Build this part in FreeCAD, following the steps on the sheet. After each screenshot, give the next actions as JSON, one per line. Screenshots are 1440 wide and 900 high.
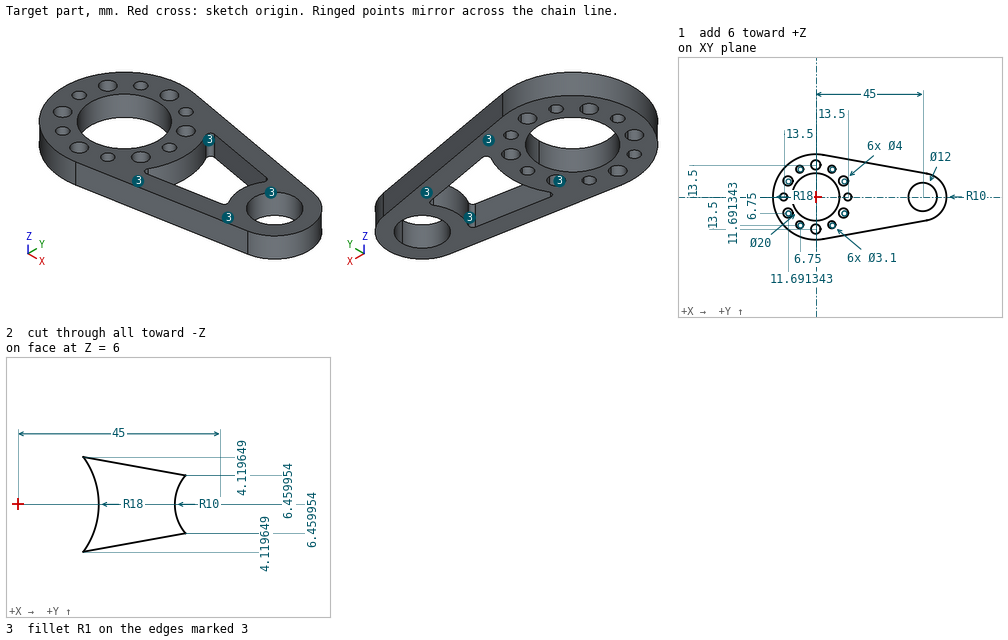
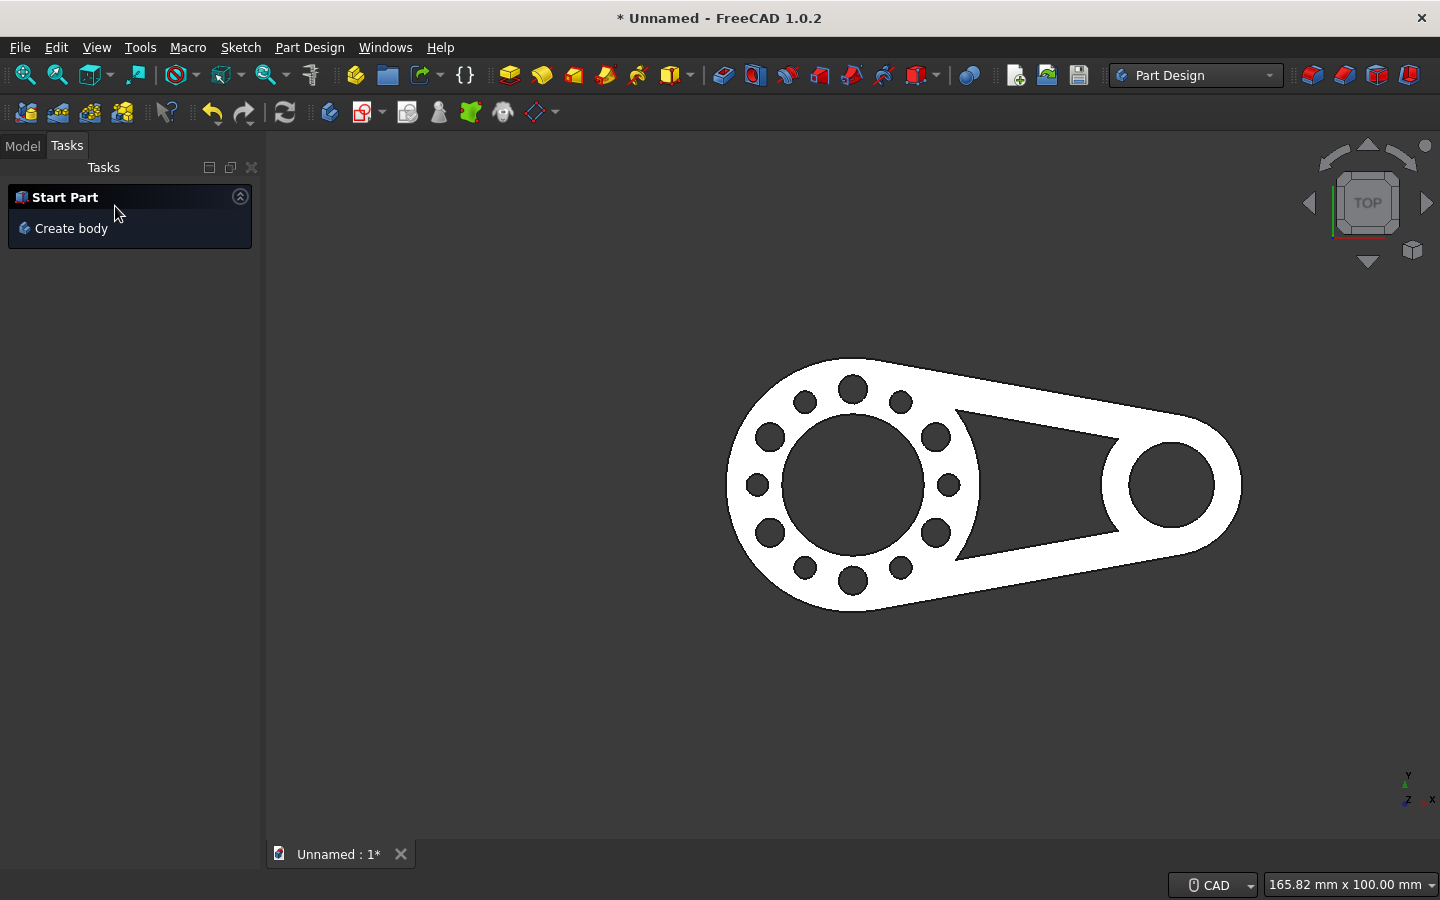
{"action": "left_click", "coordinate": [26, 76]}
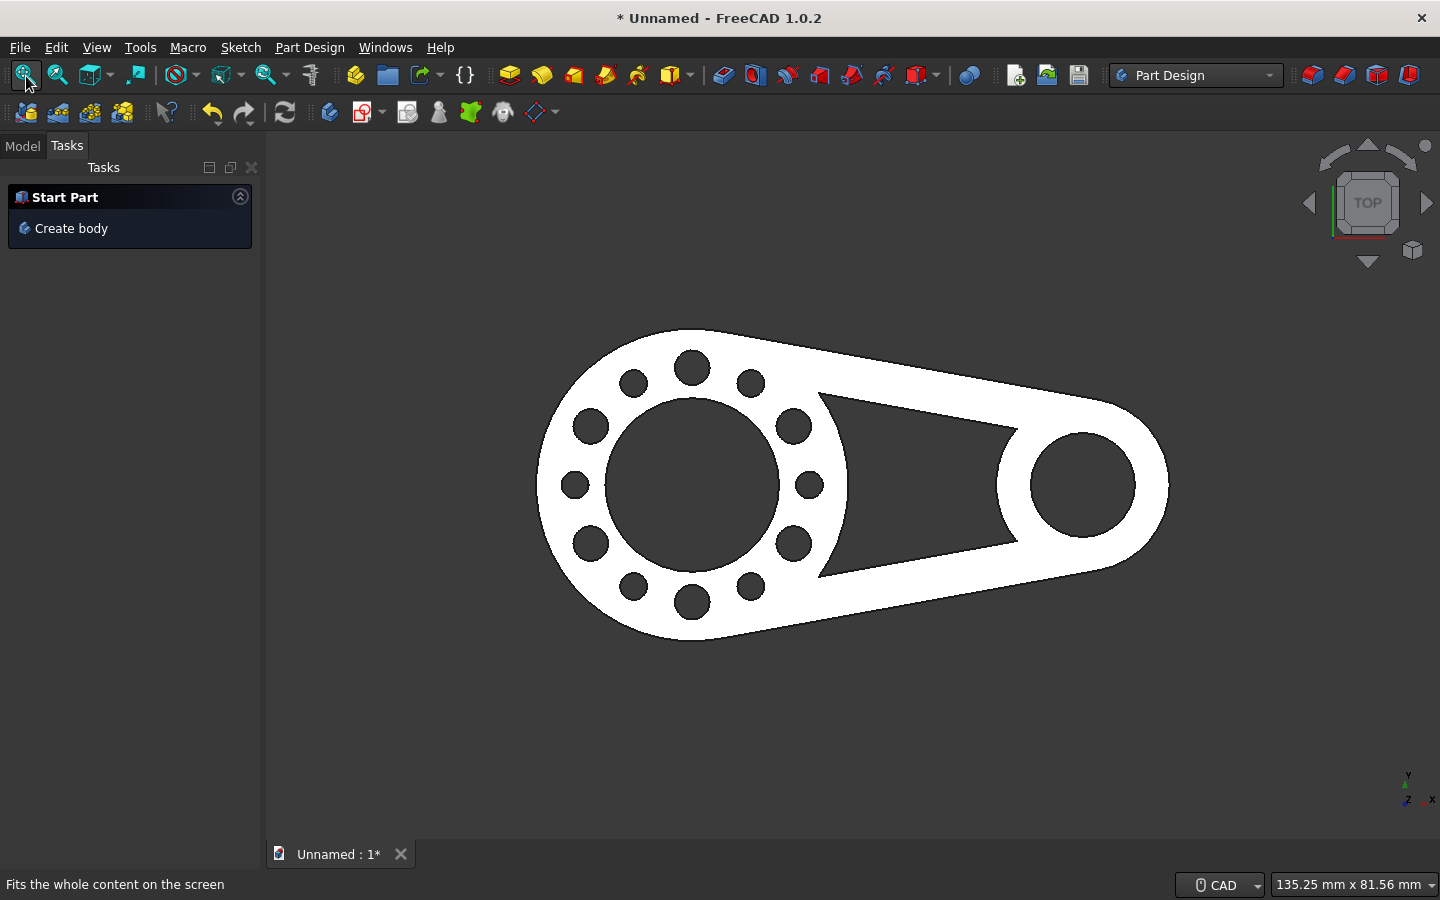
{"action": "key", "text": "1"}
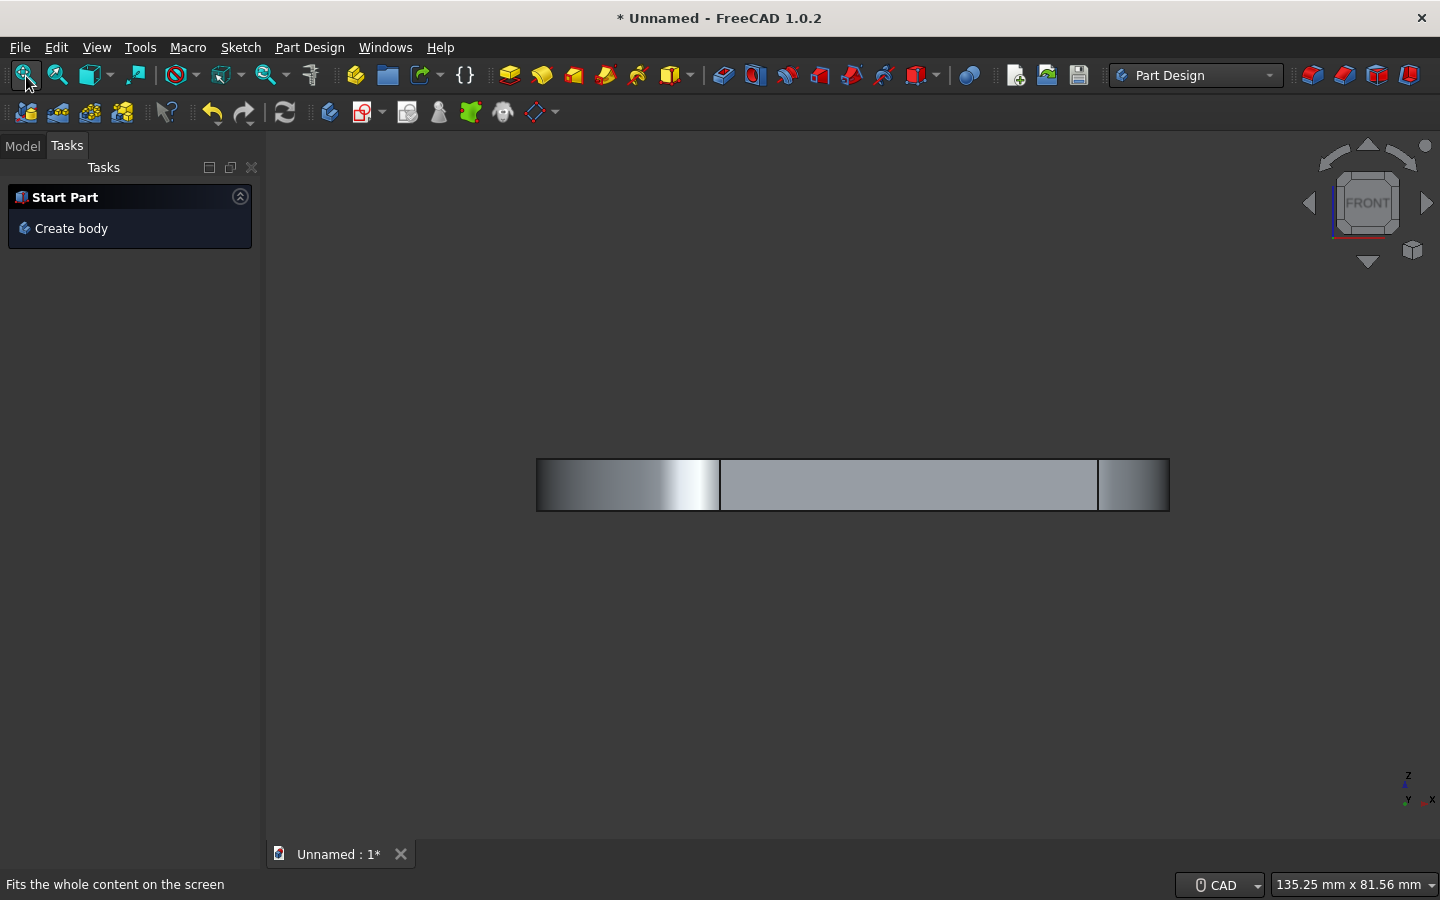
{"action": "key", "text": "3"}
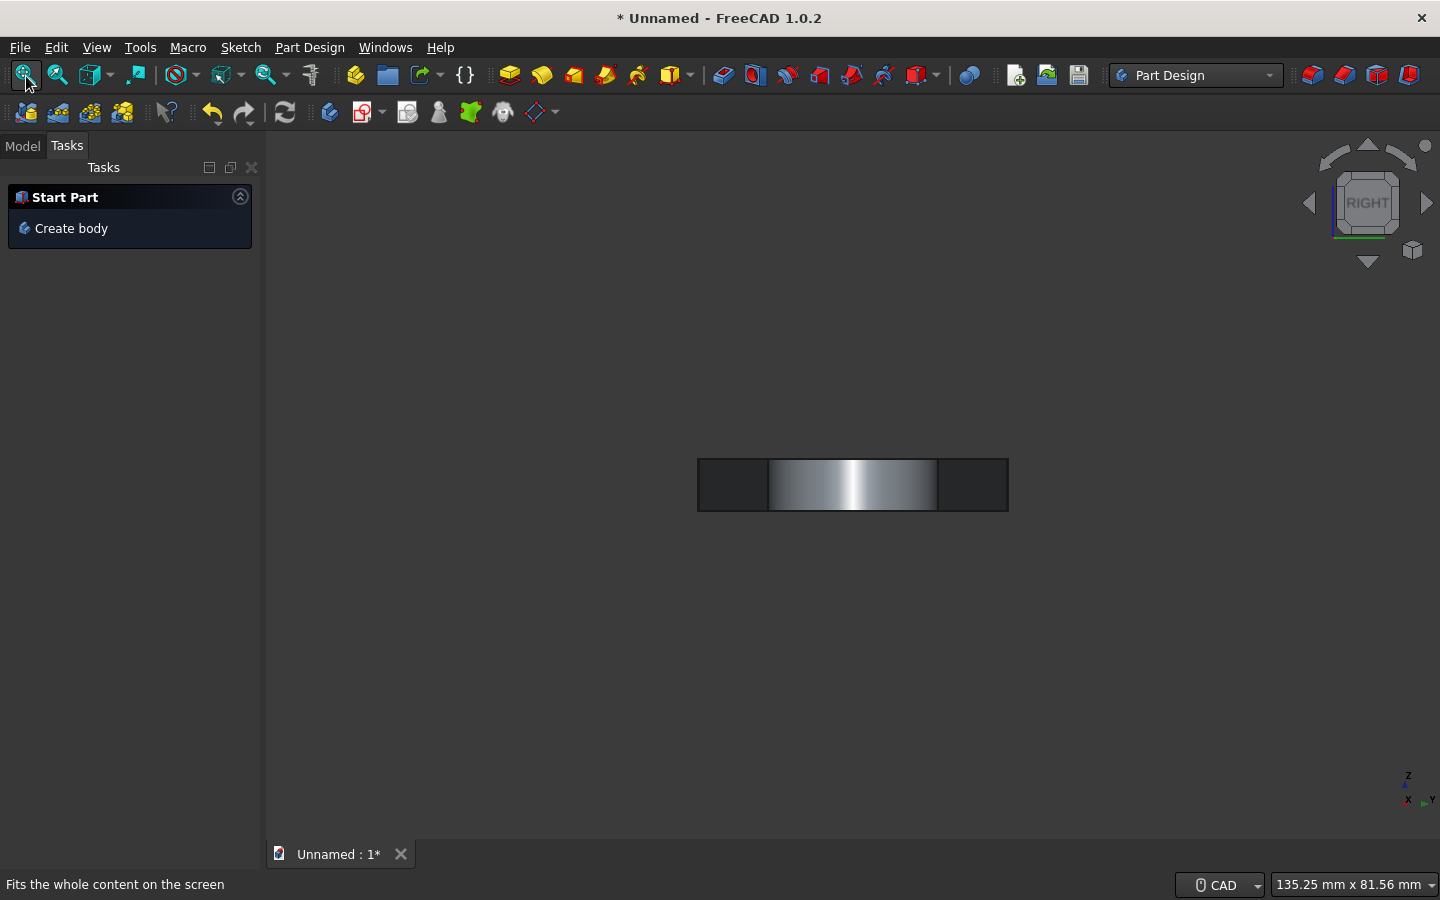
{"action": "left_click", "coordinate": [26, 76]}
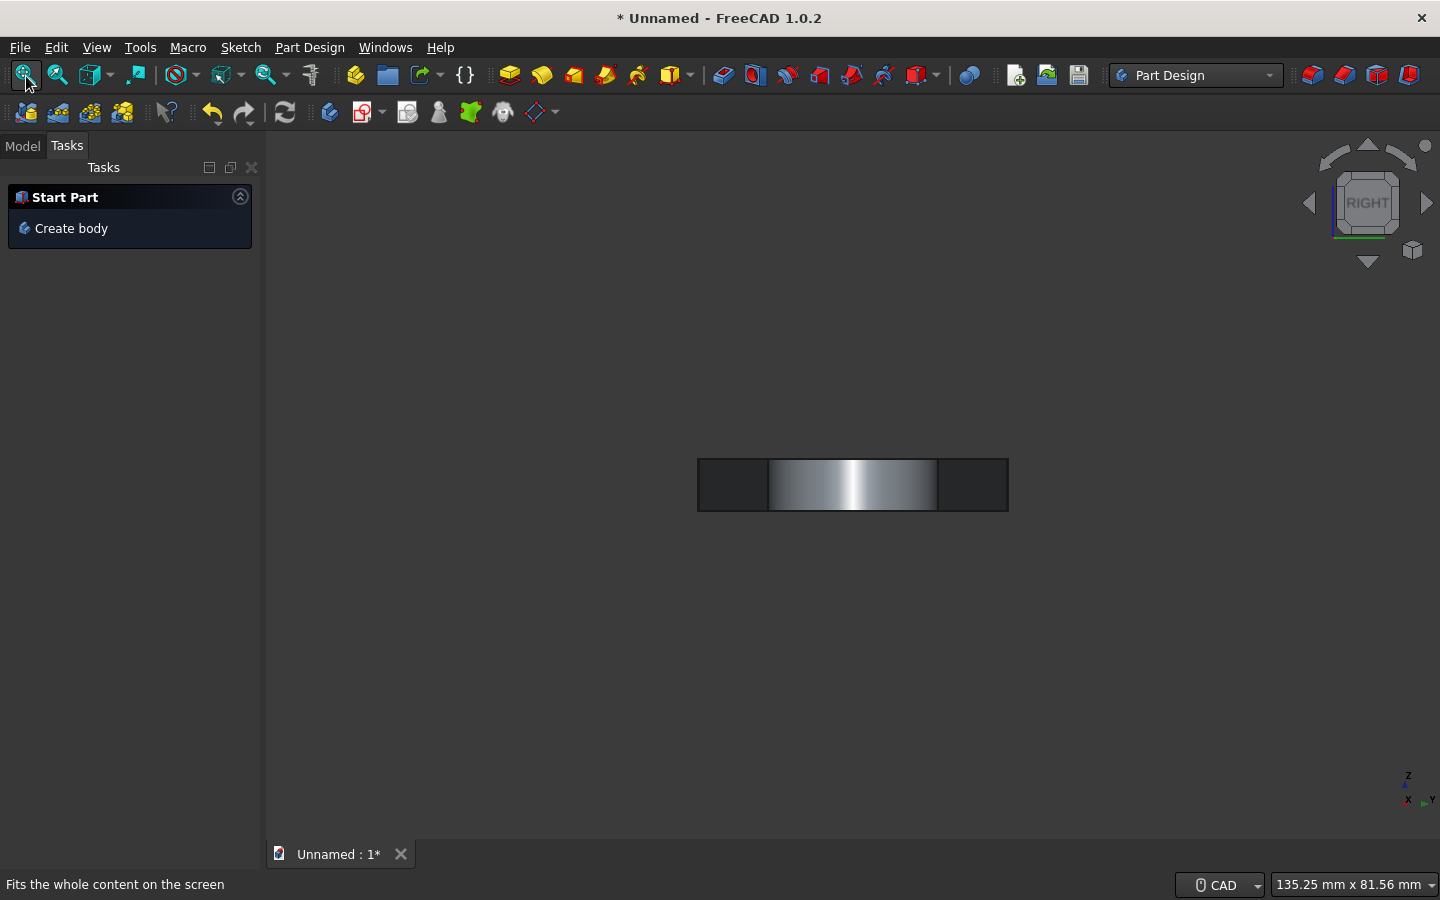
{"action": "key", "text": "5"}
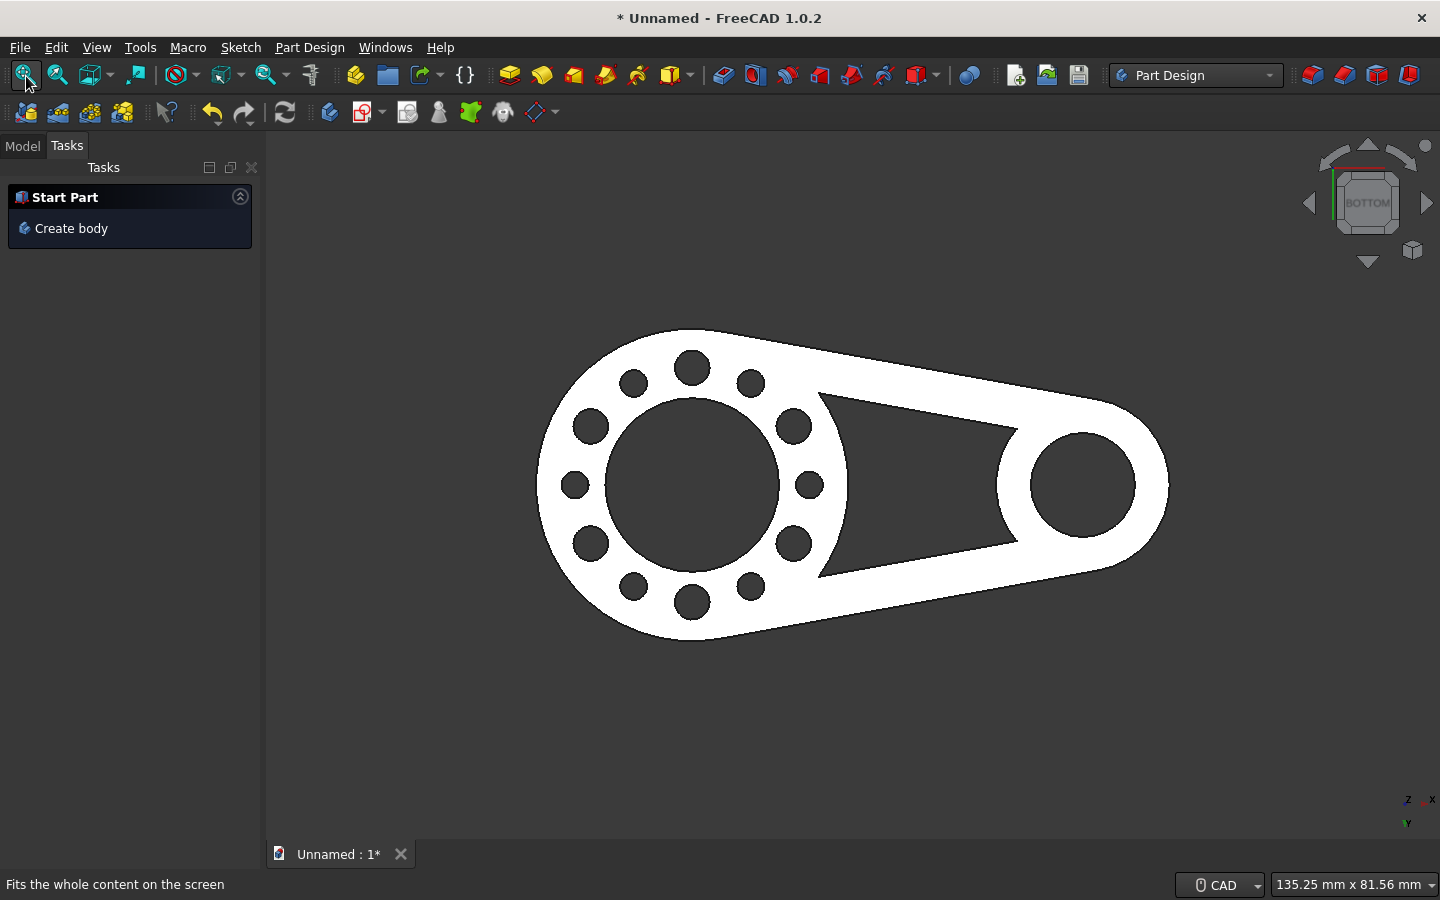
{"action": "key", "text": "4"}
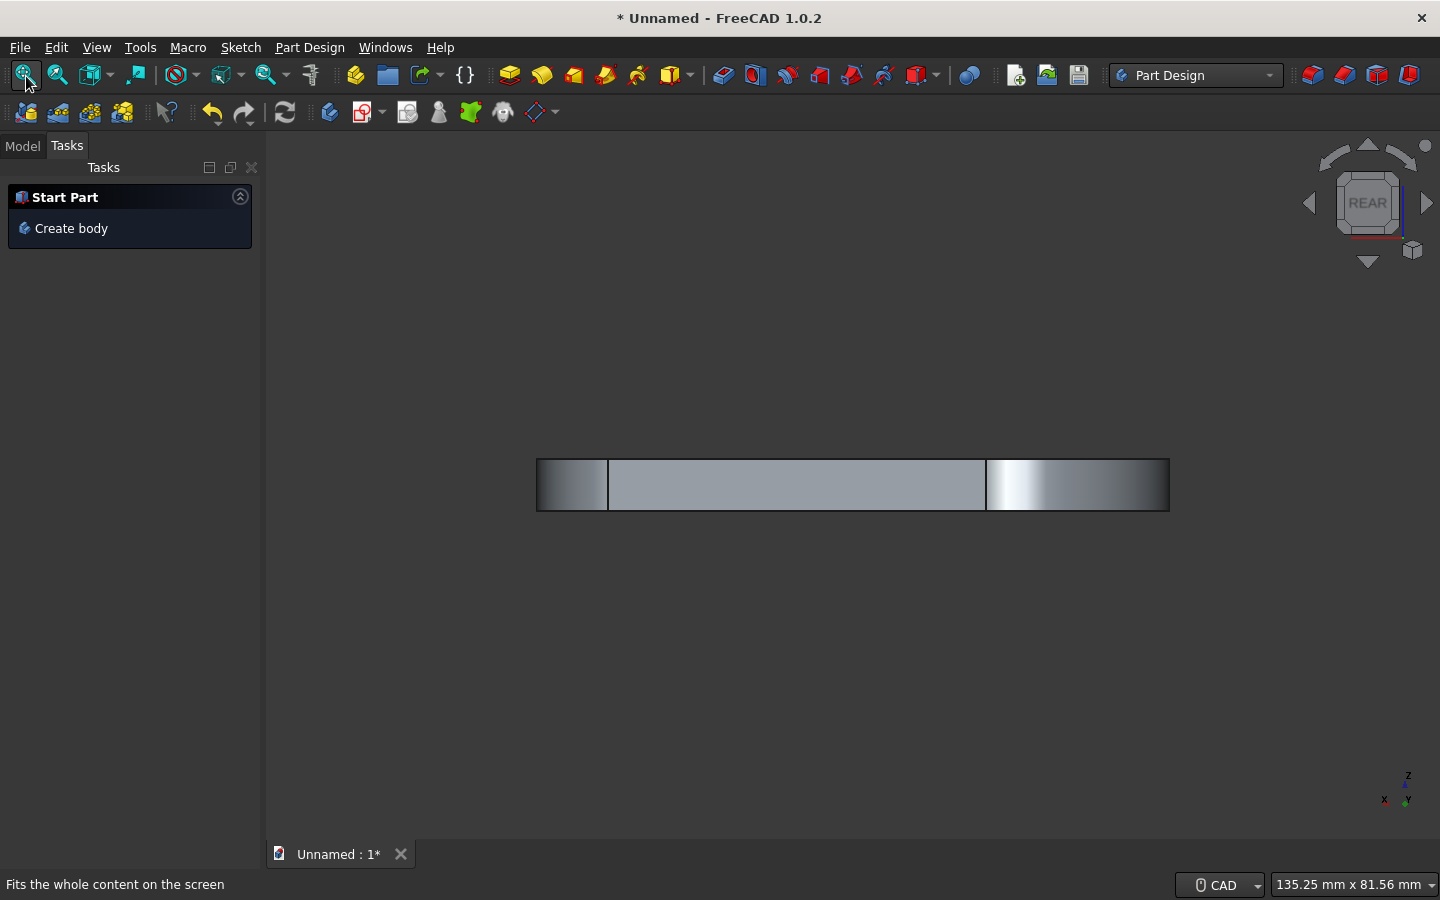
{"action": "key", "text": "6"}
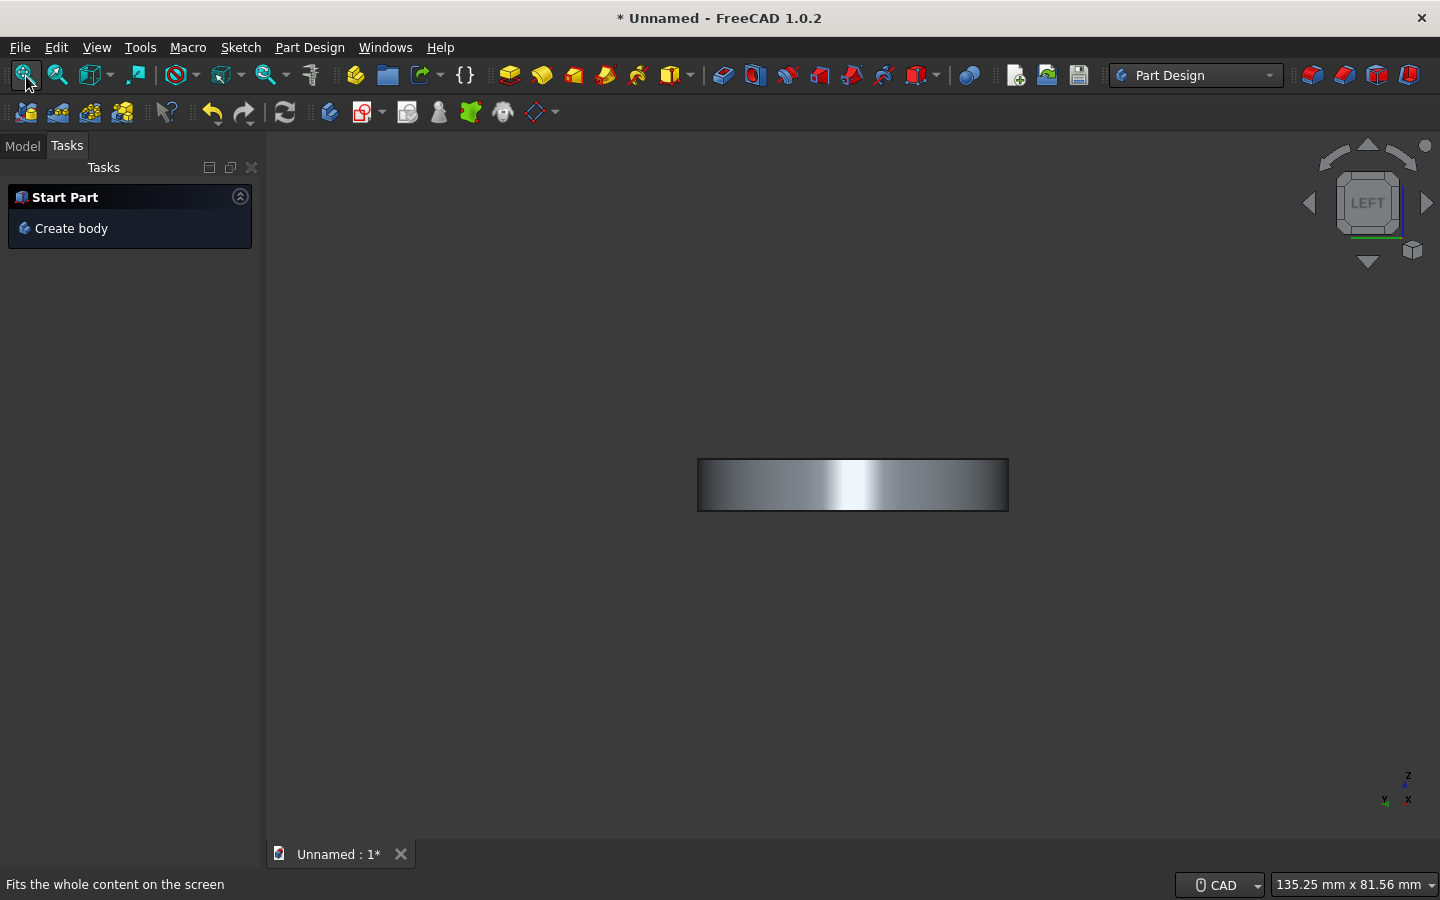
{"action": "left_click", "coordinate": [26, 76]}